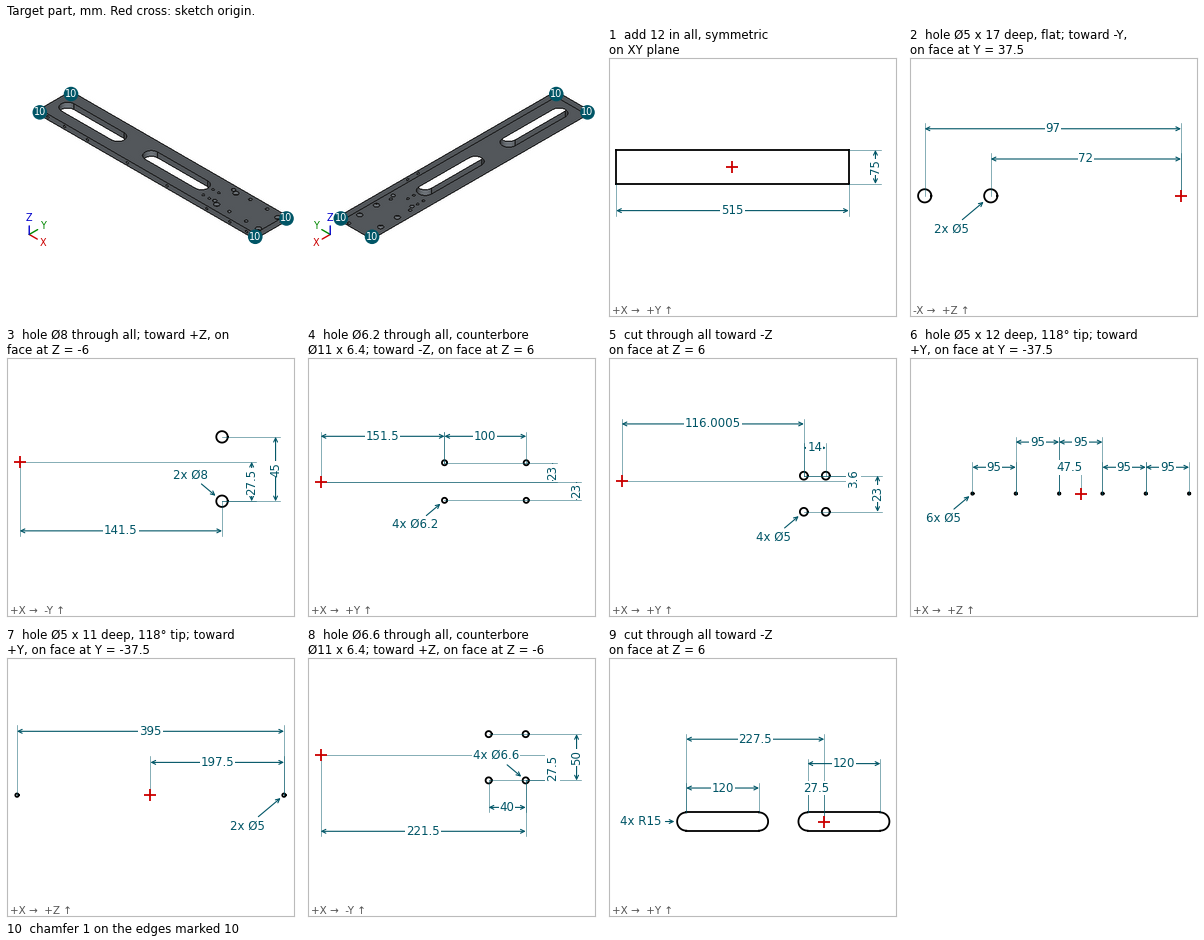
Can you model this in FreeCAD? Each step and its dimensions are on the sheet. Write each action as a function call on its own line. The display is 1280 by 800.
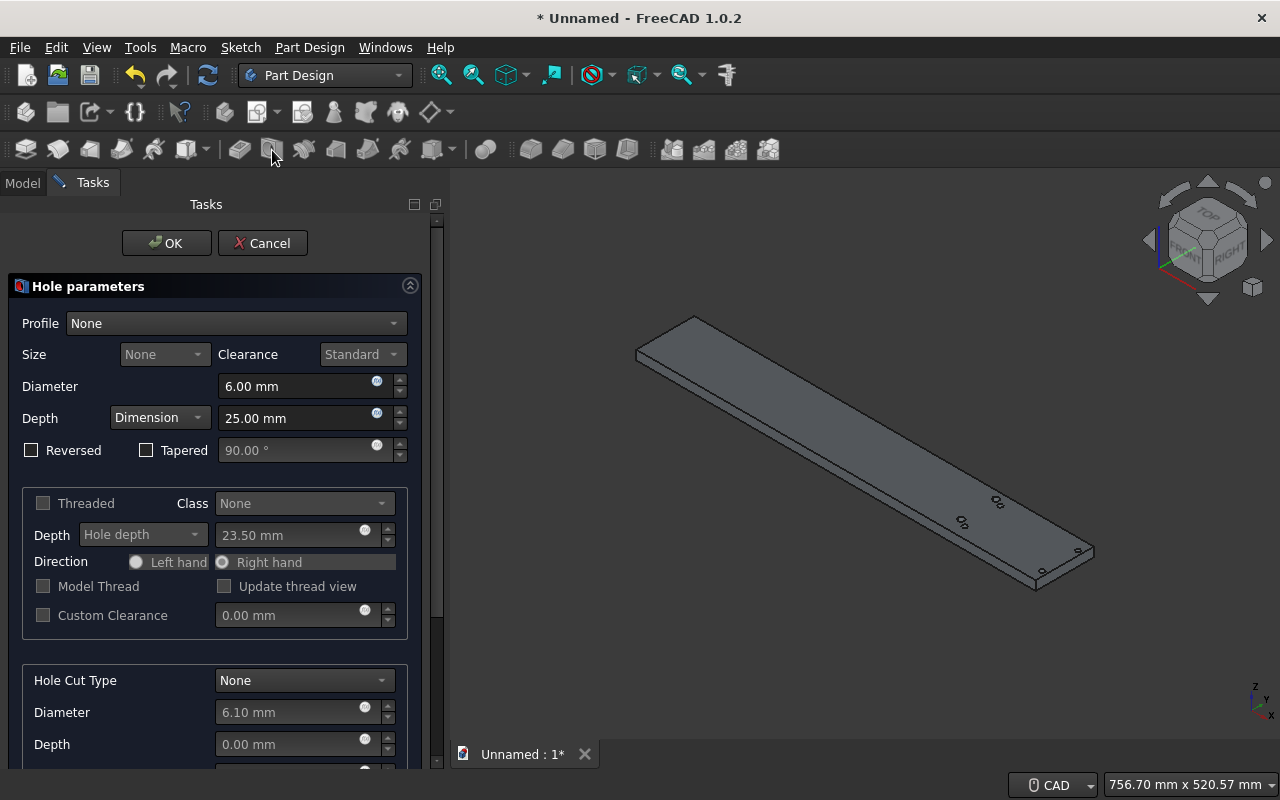
triple_click(305, 386)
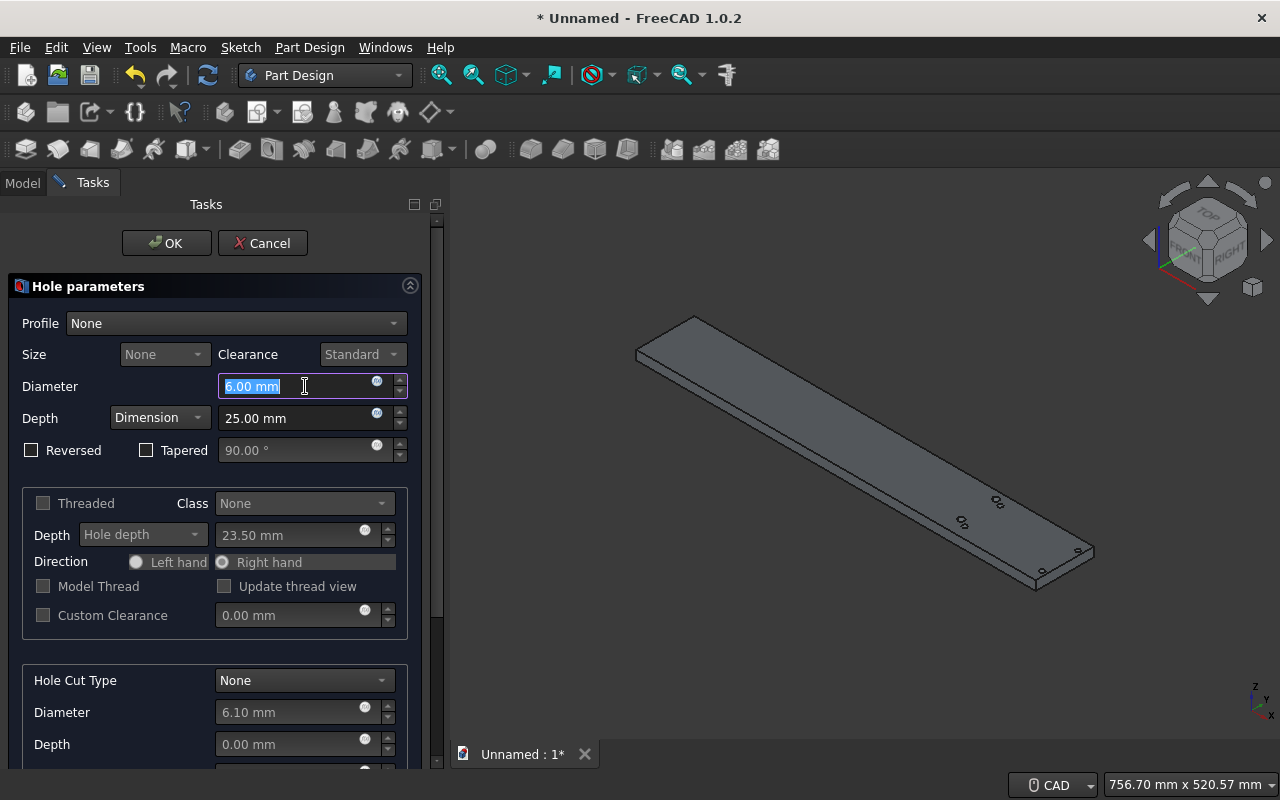
text(6.2)
key(Tab)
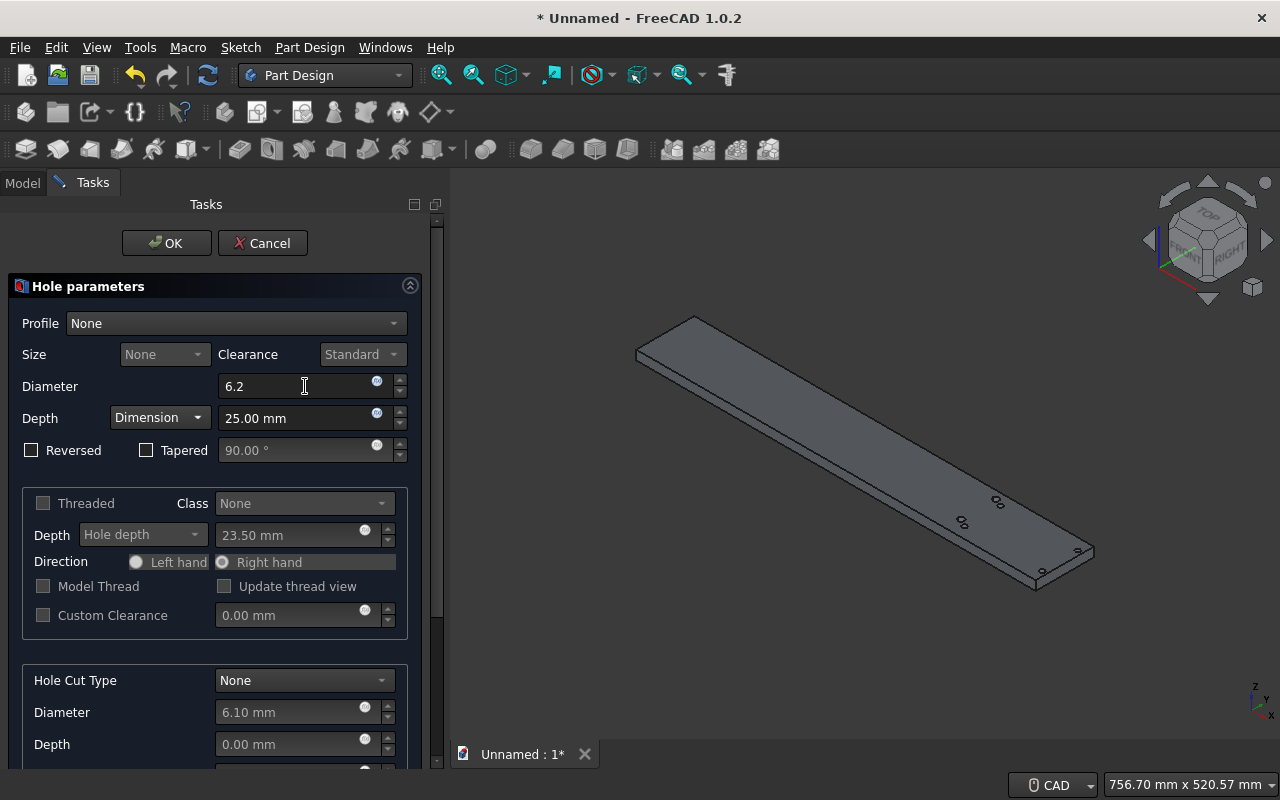
click(161, 418)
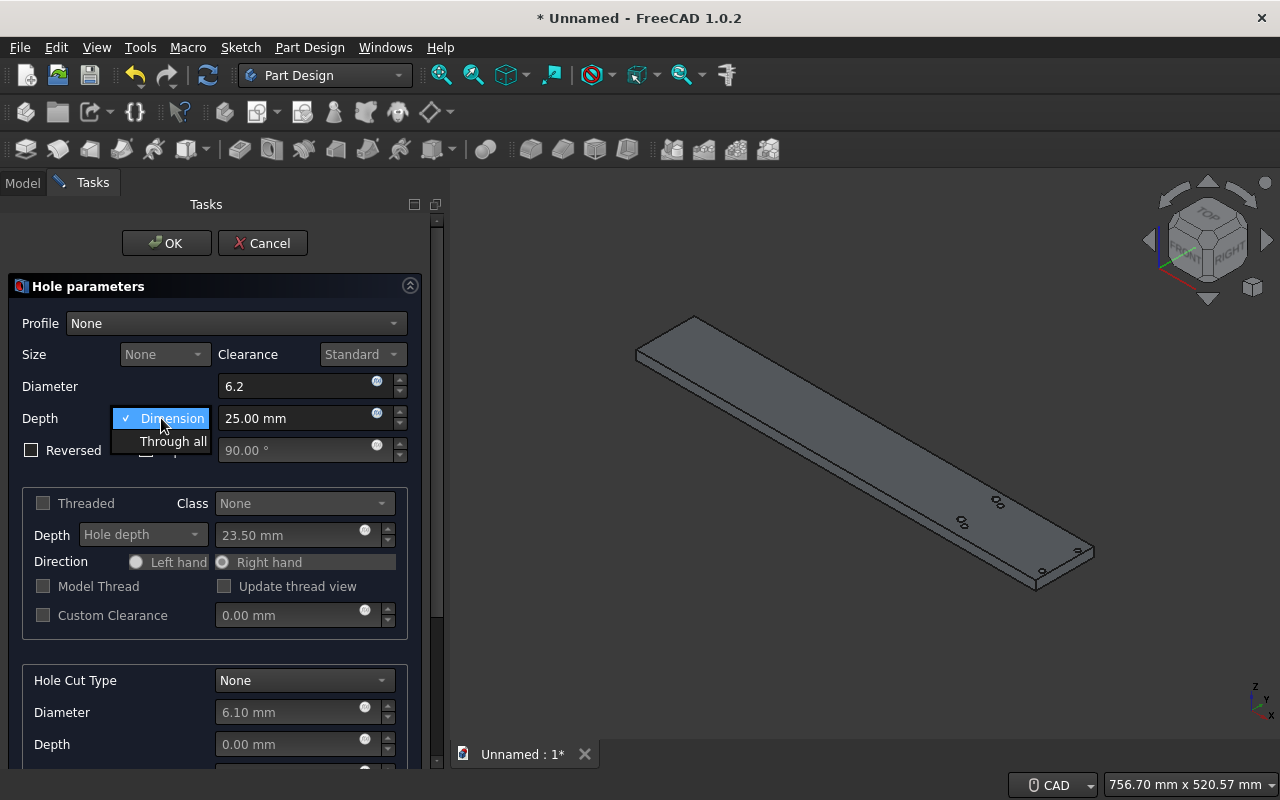
click(160, 442)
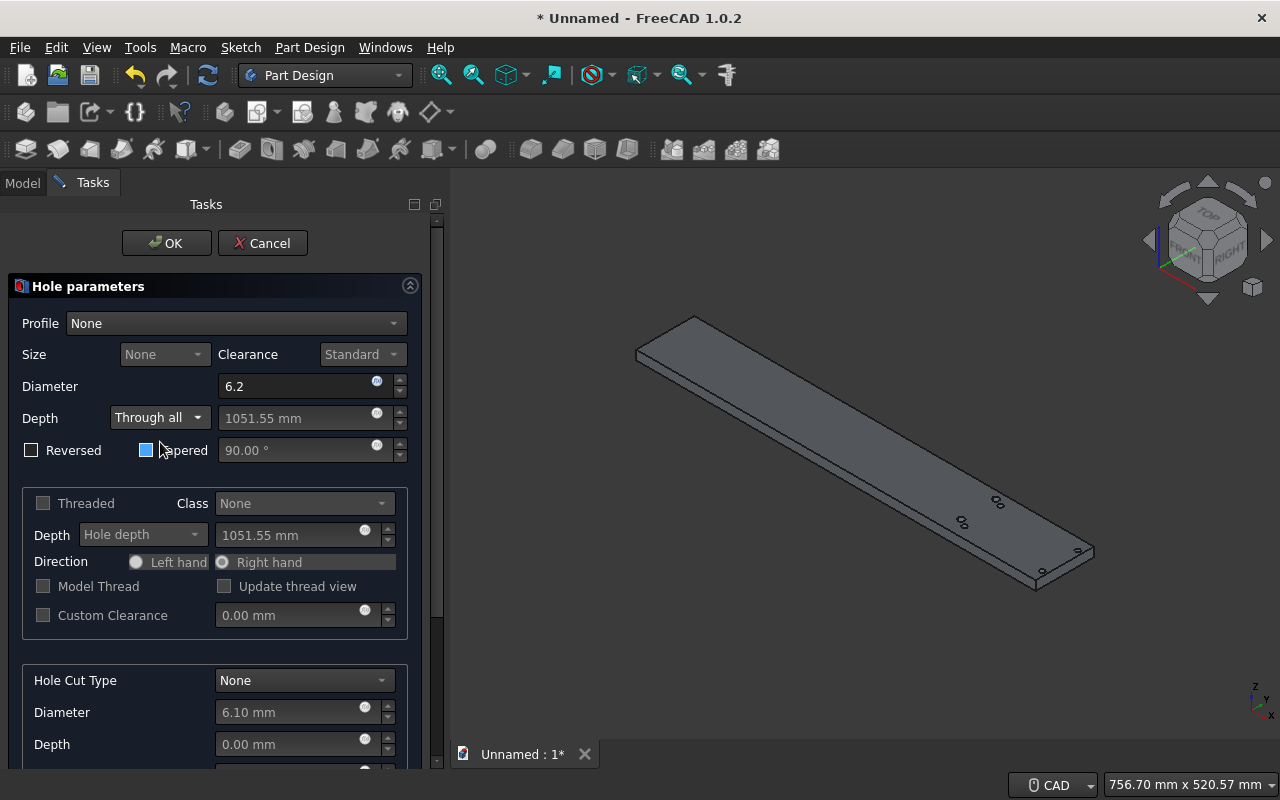
click(306, 680)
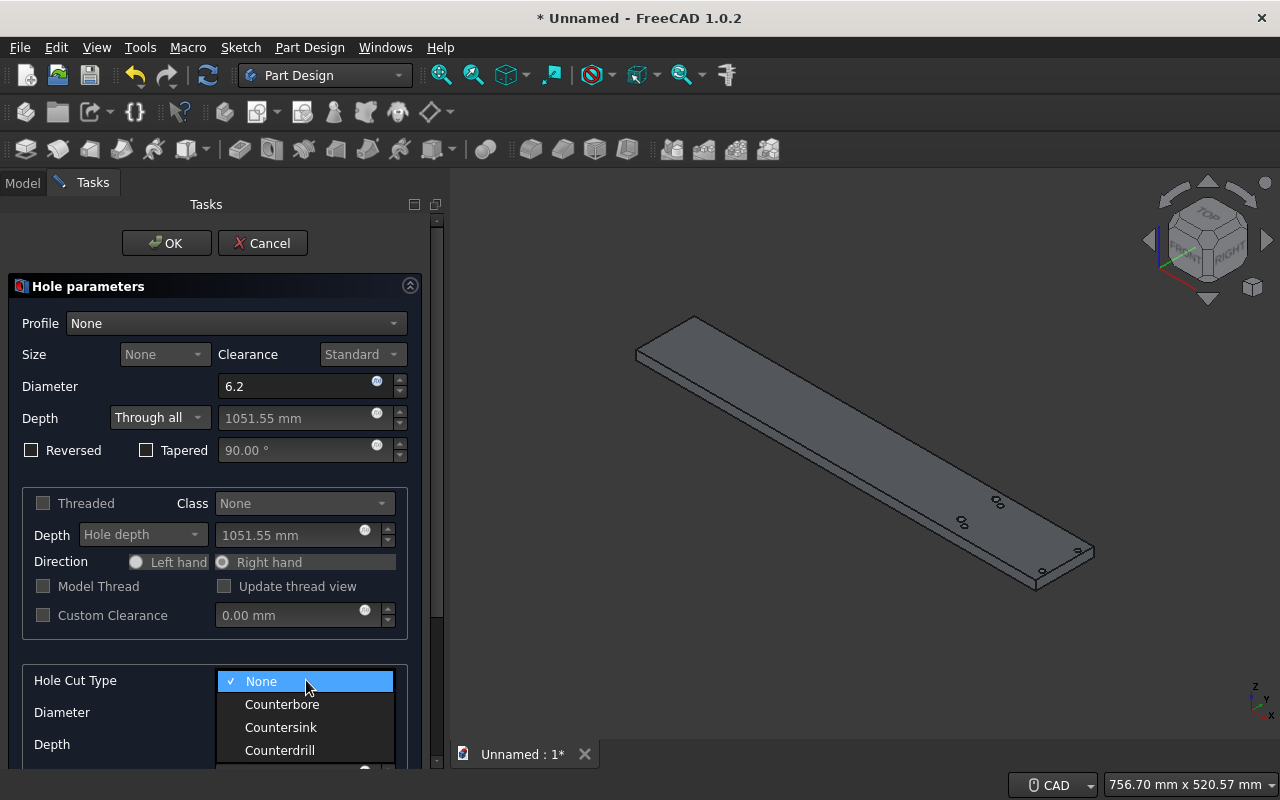
click(304, 704)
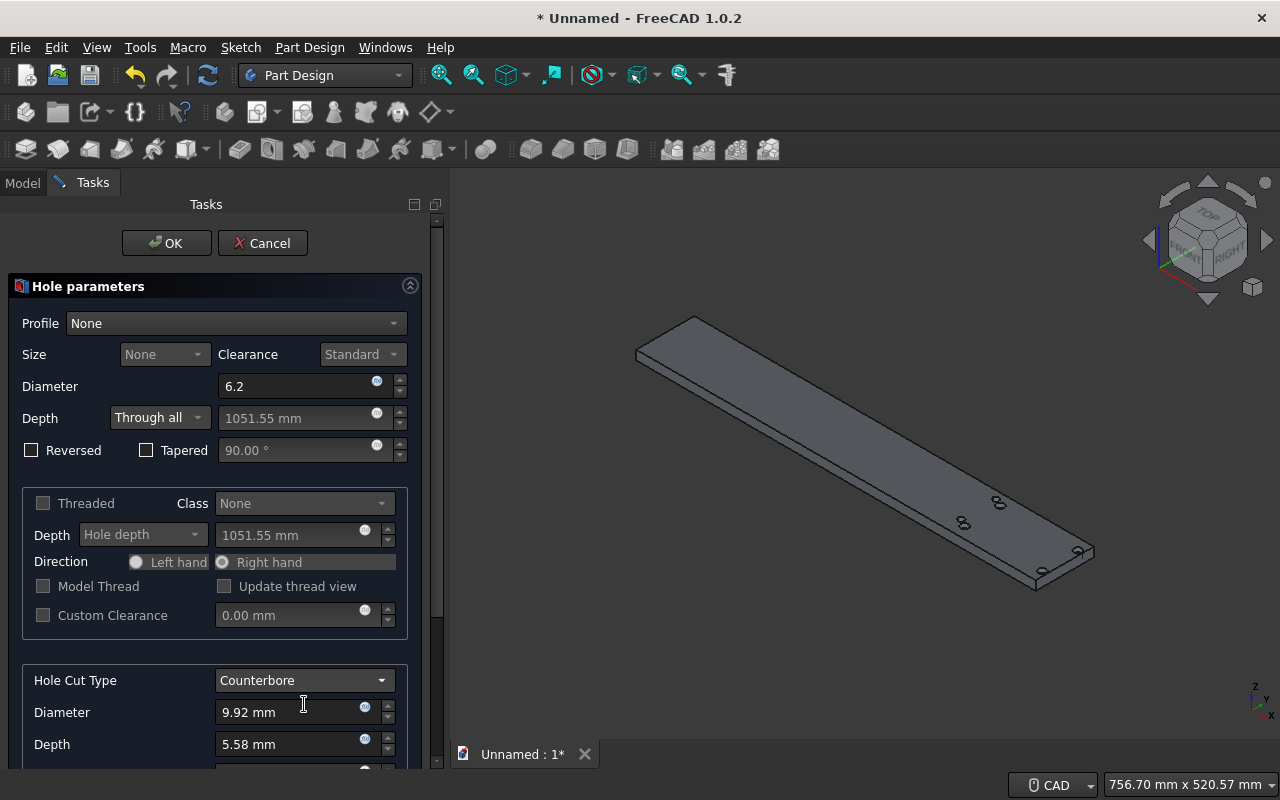
triple_click(298, 712)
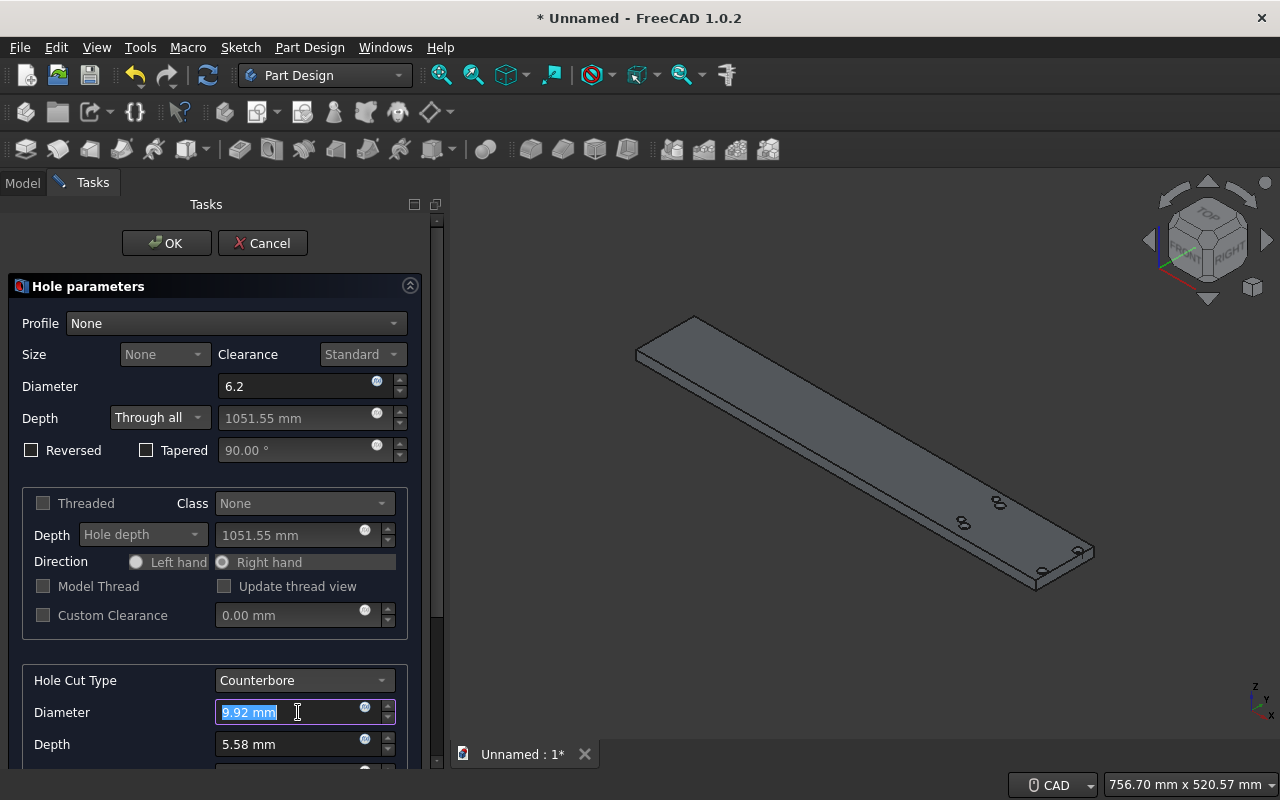
text(11)
key(Tab)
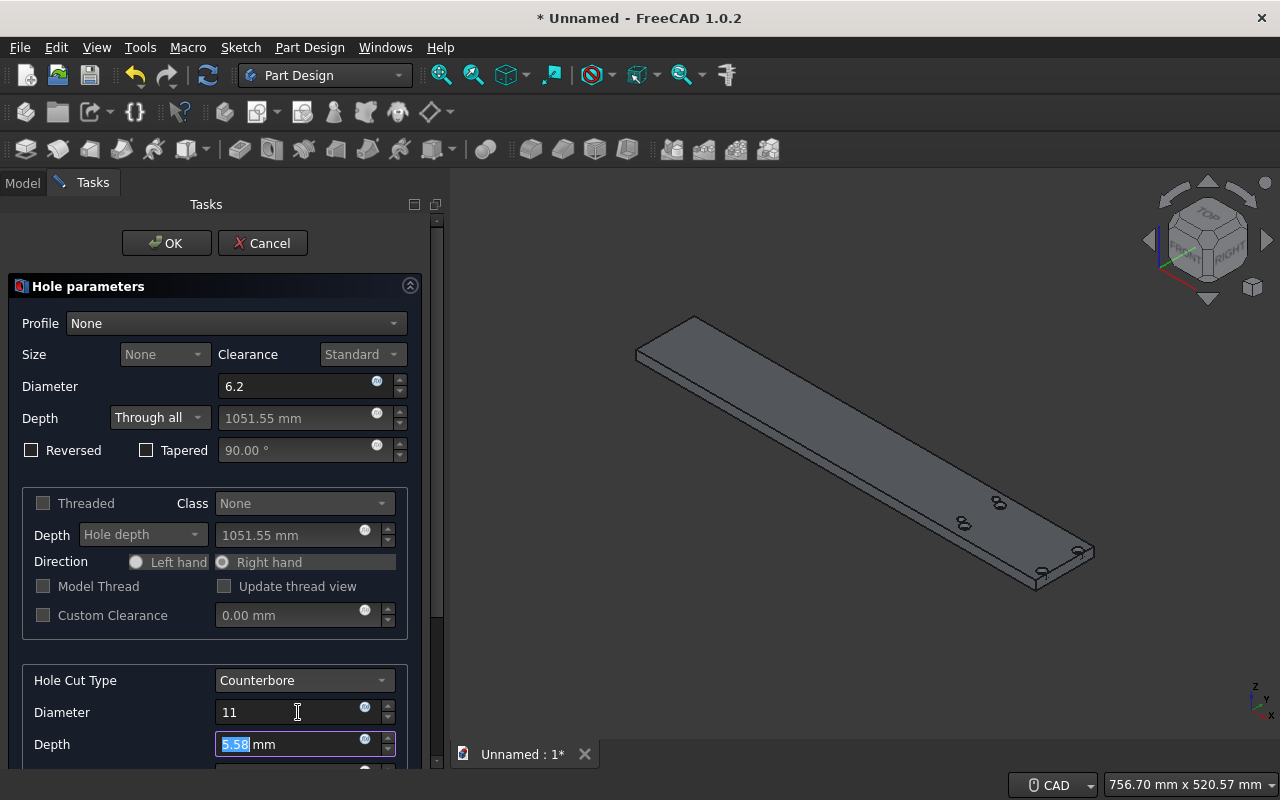
text(6.4)
key(Tab)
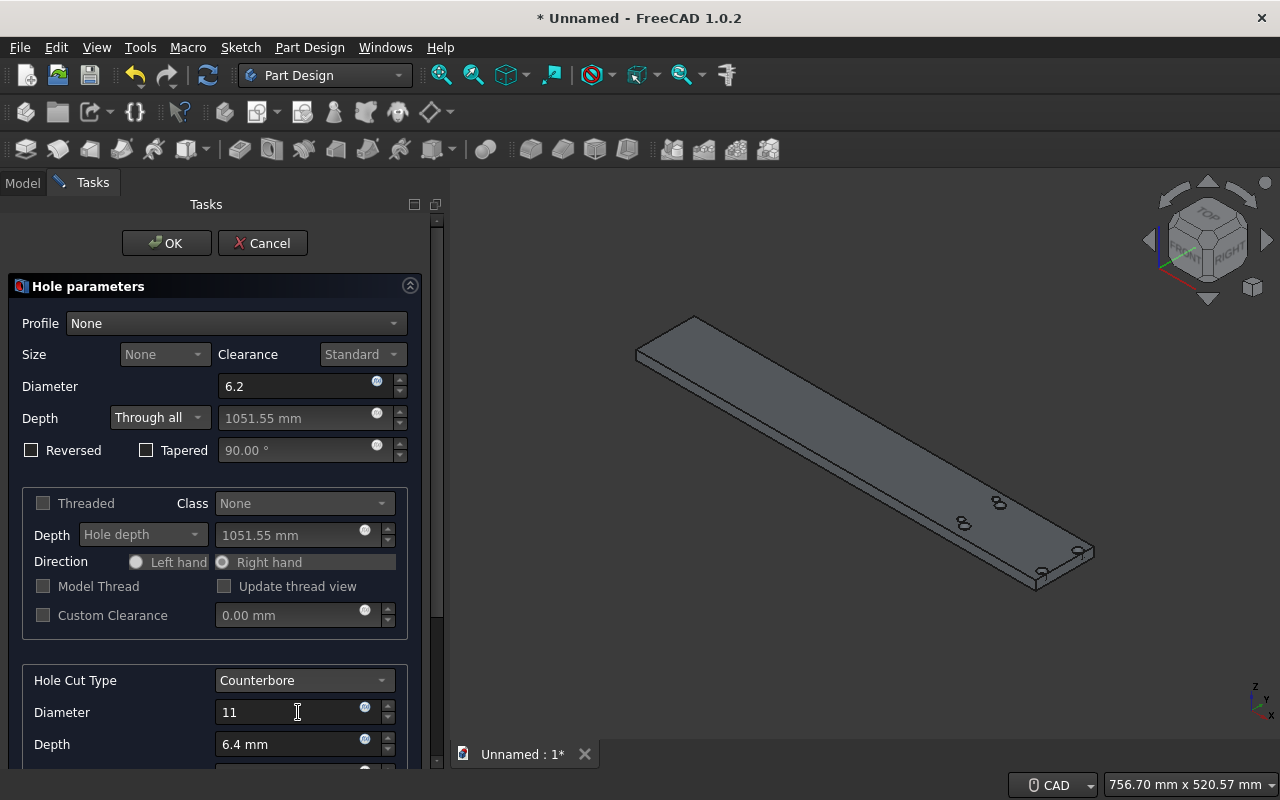
click(167, 243)